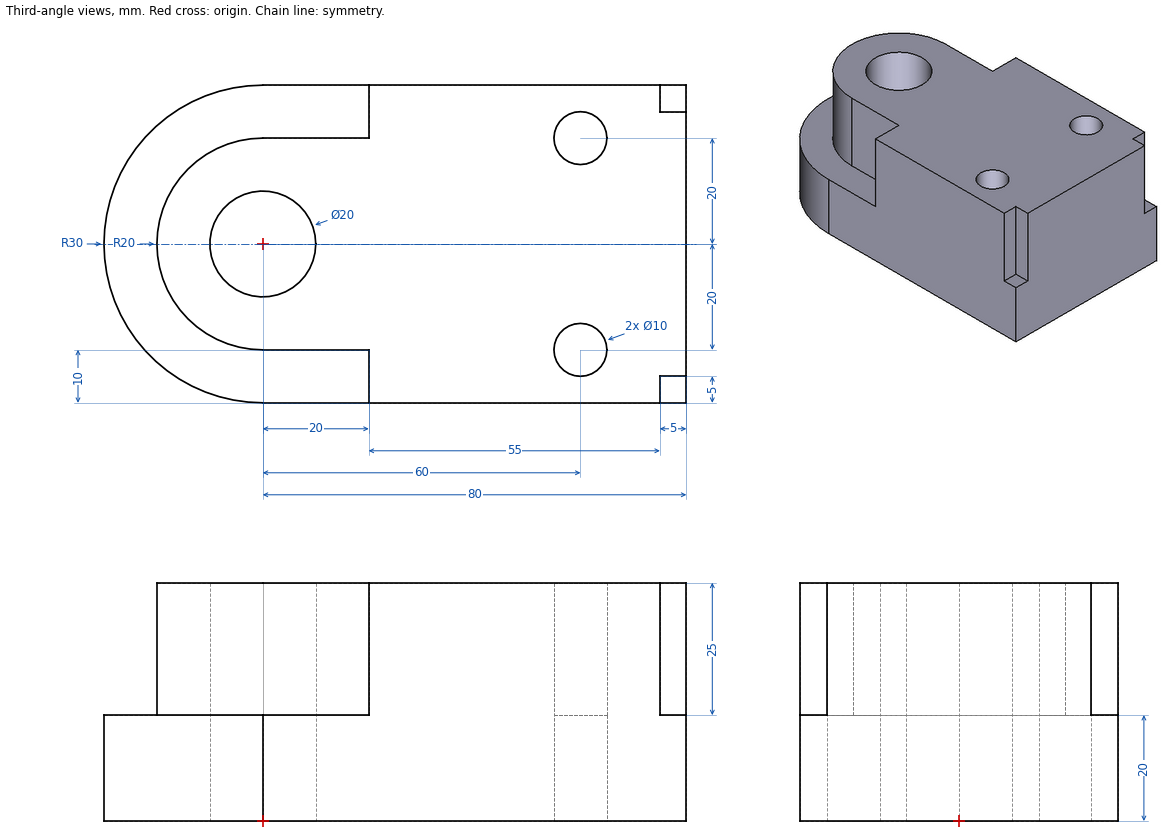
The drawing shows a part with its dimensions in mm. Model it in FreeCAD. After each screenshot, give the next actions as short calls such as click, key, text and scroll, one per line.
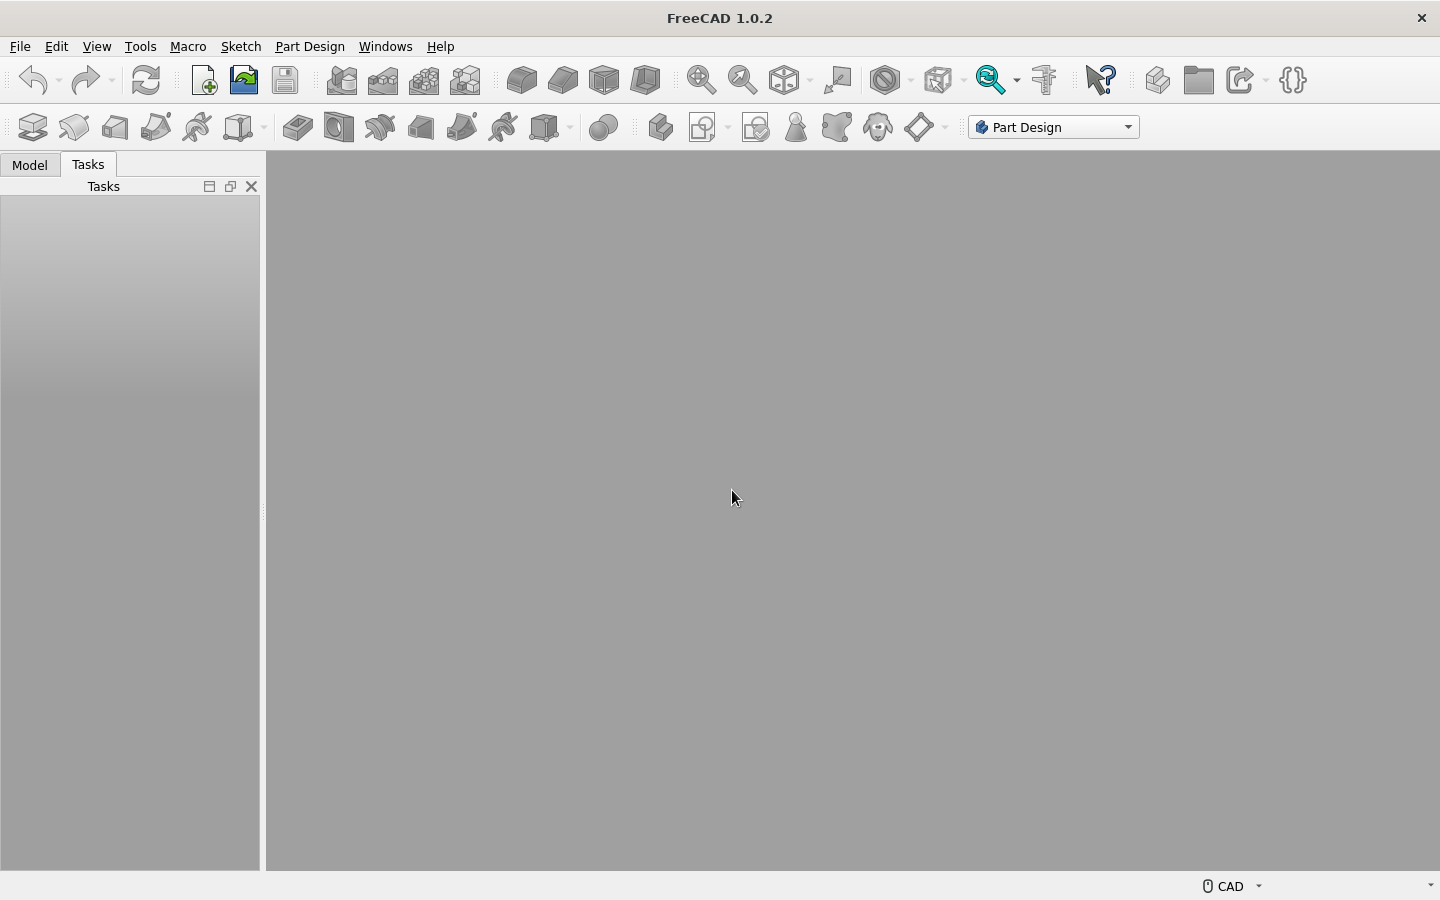
key(ctrl+n)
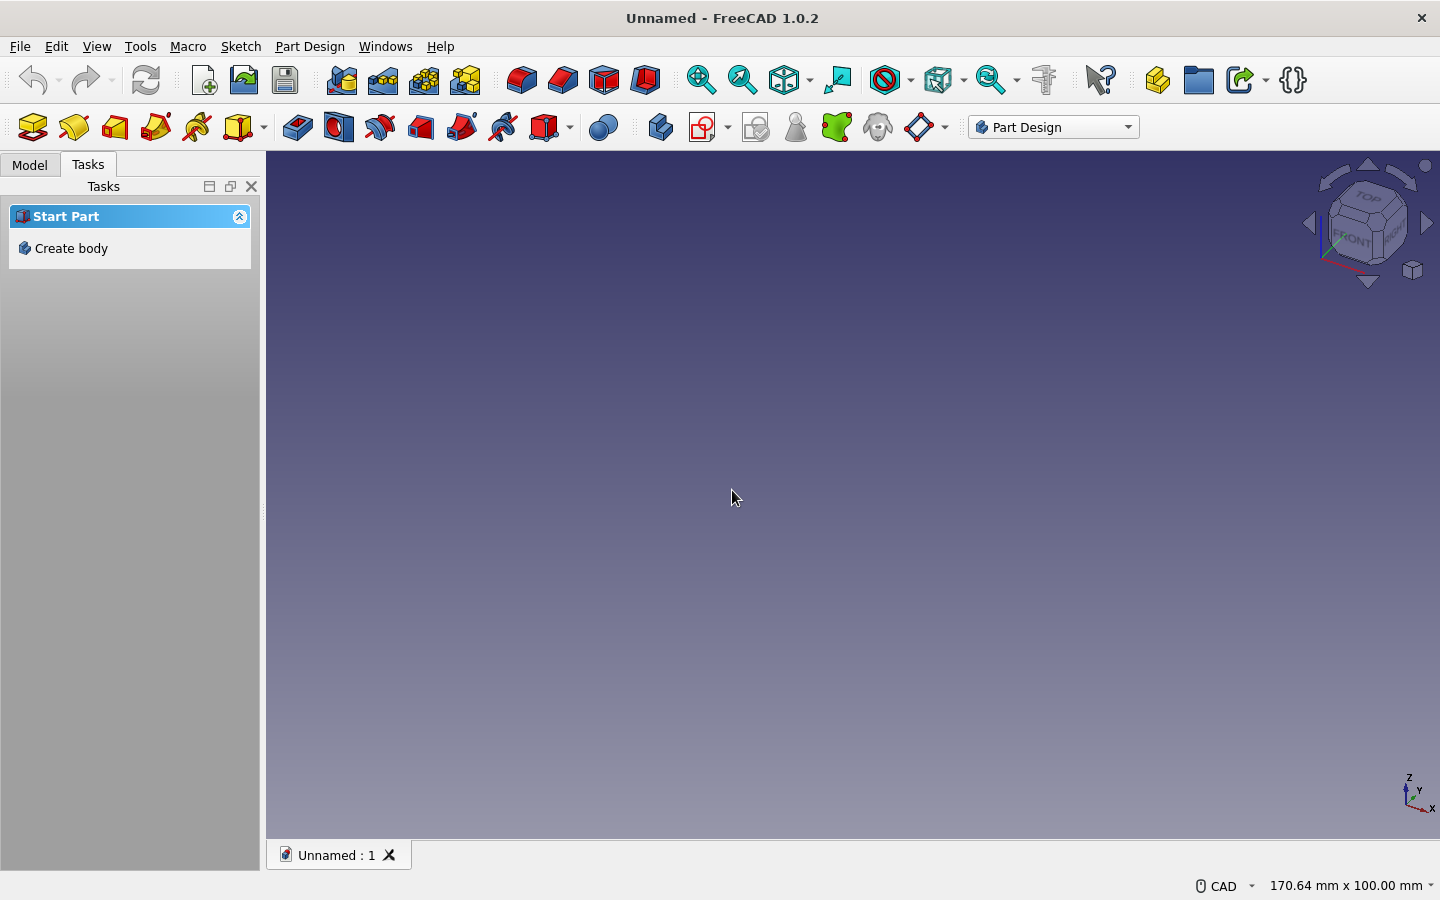
click(702, 128)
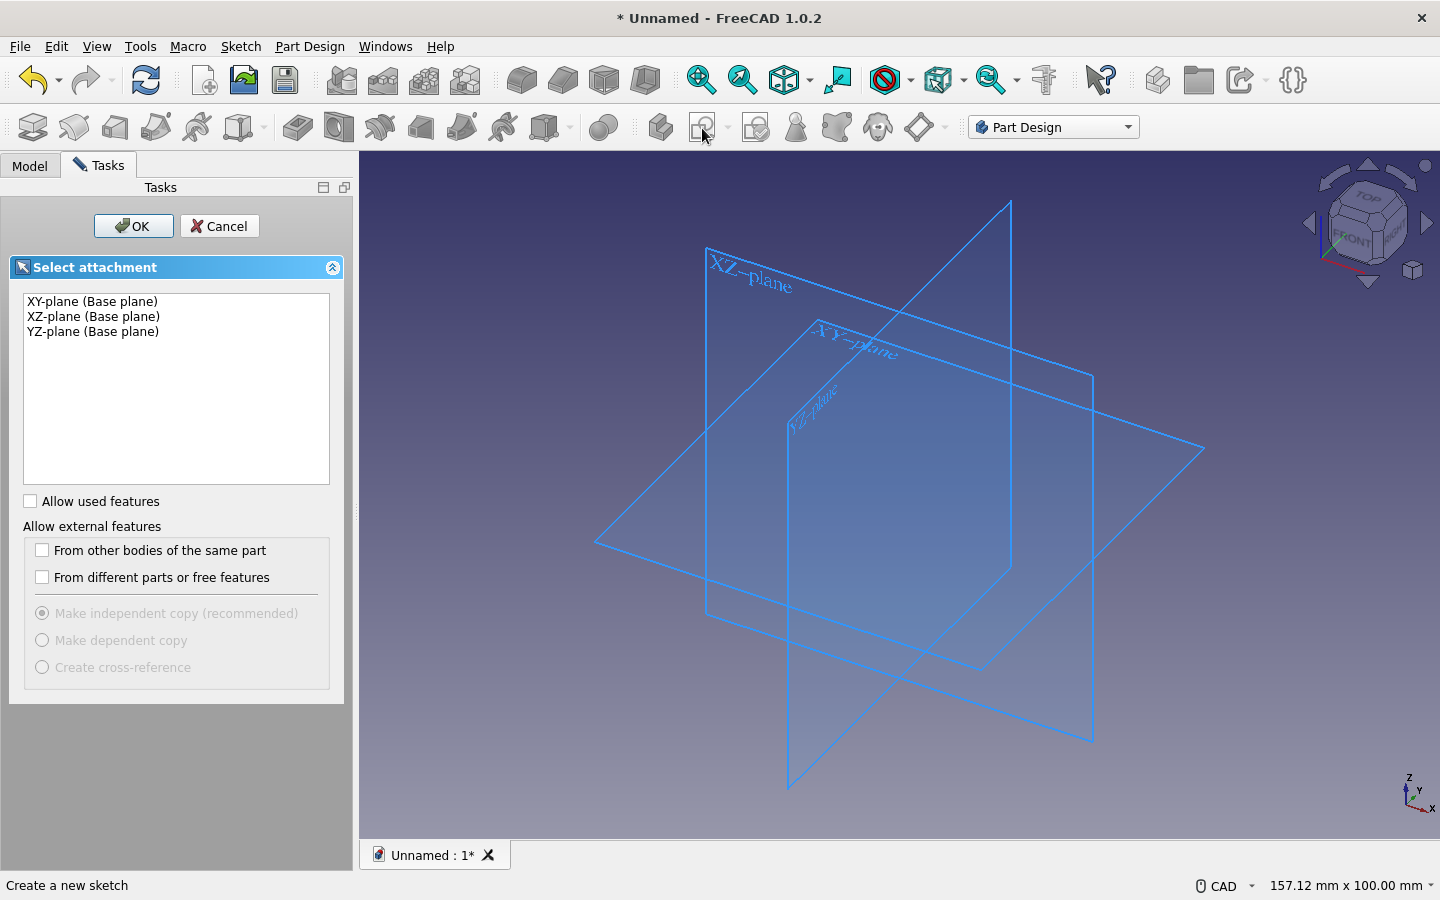
click(84, 302)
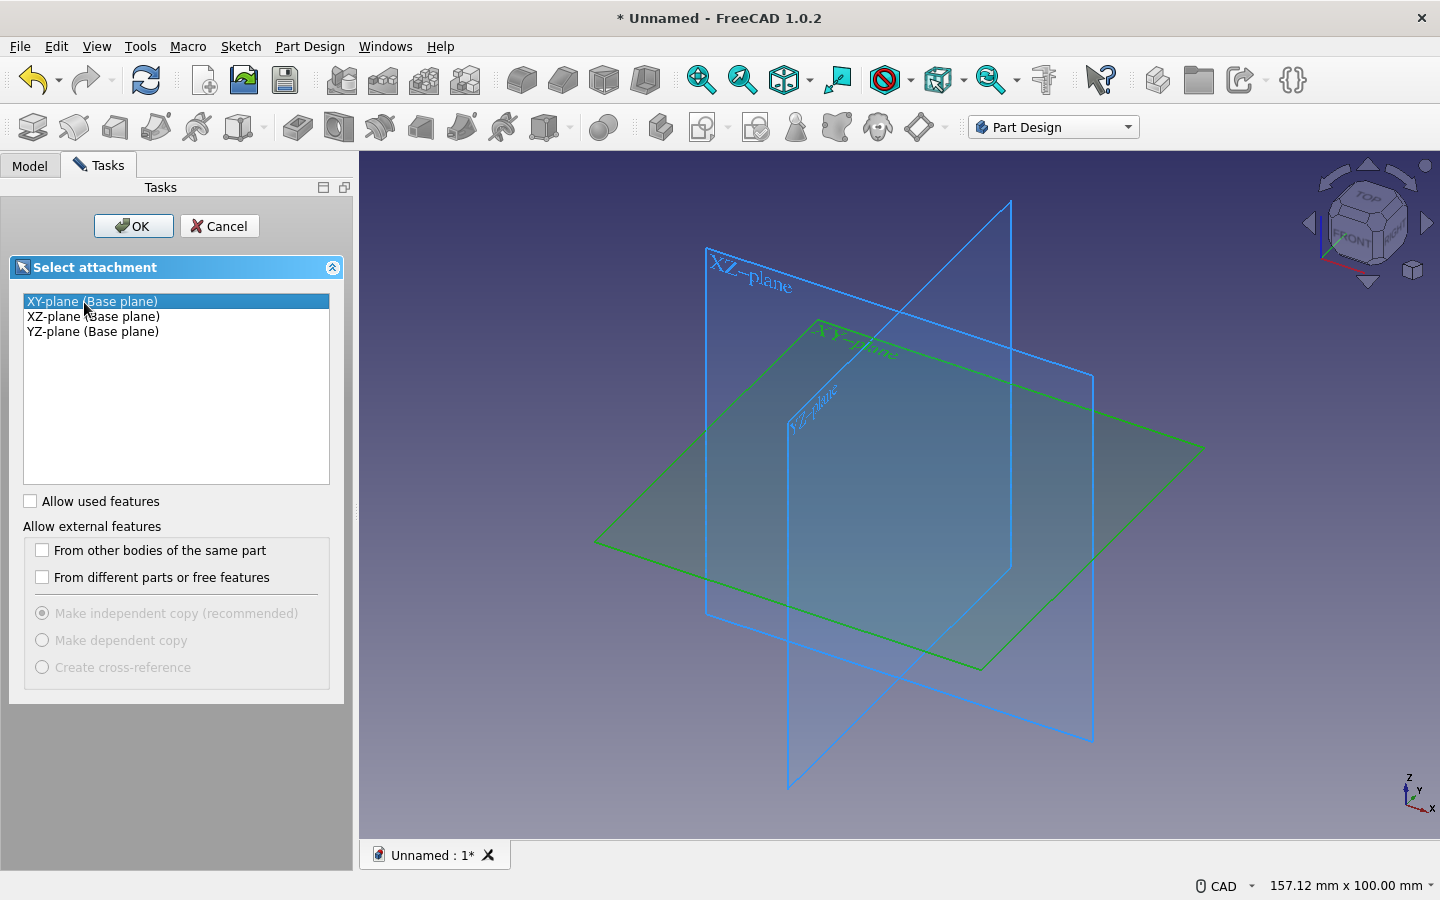
click(134, 226)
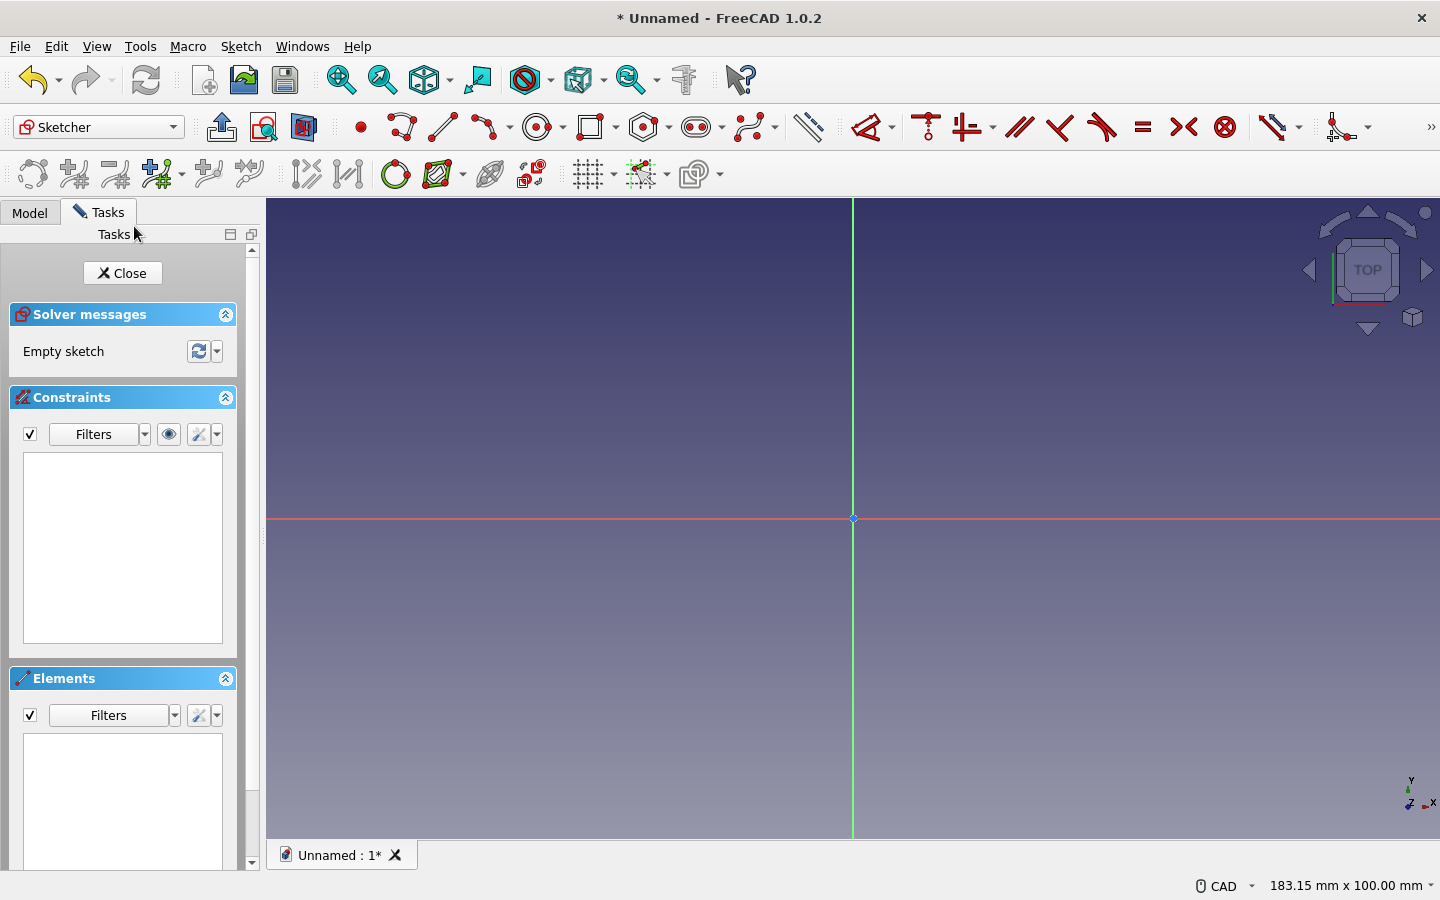
scroll(294, 519, down, 1)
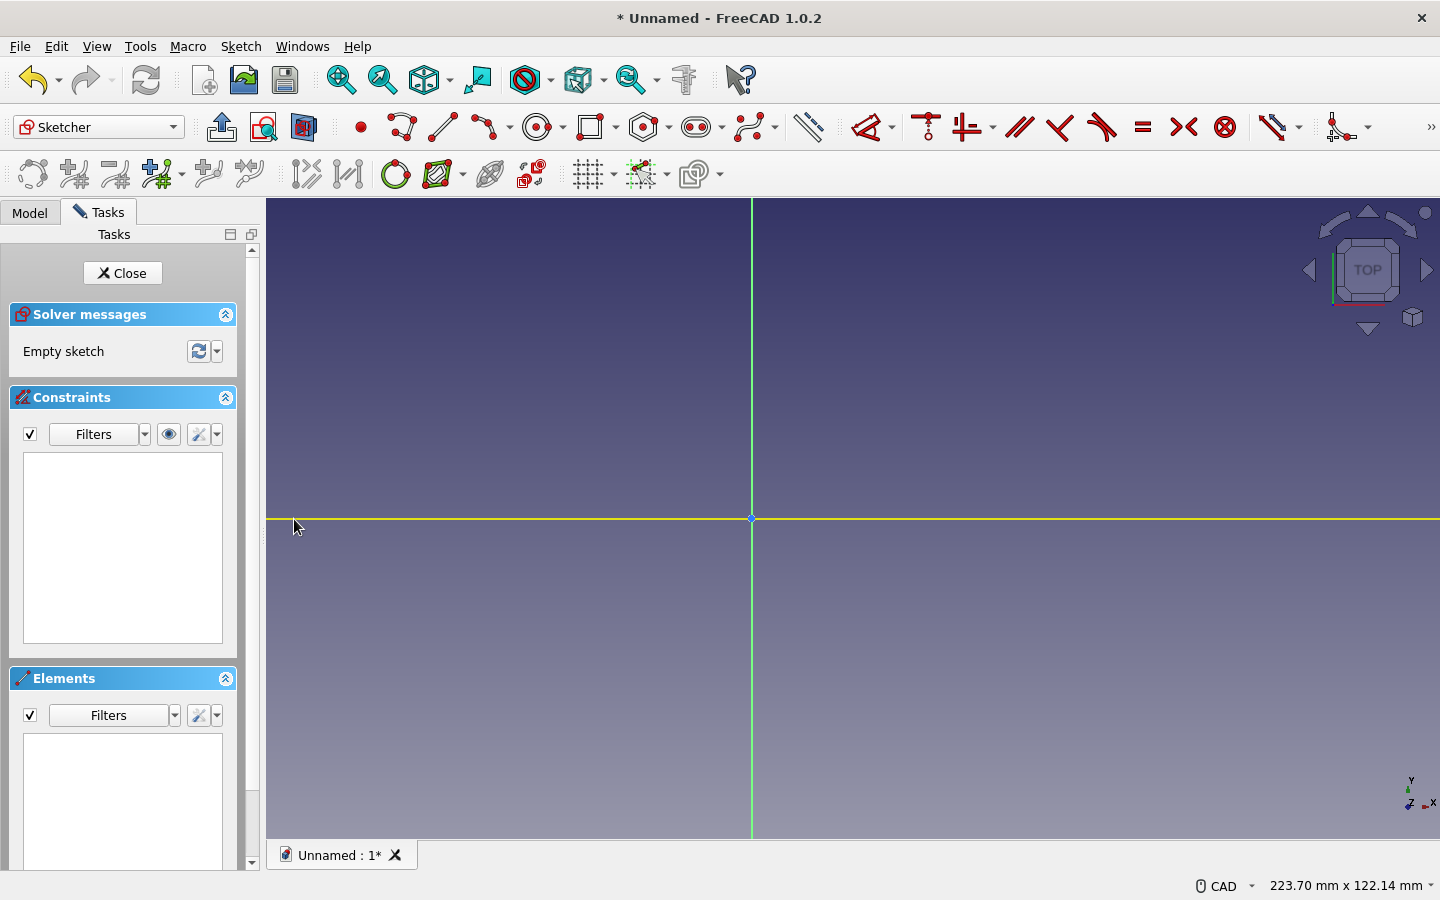
click(402, 128)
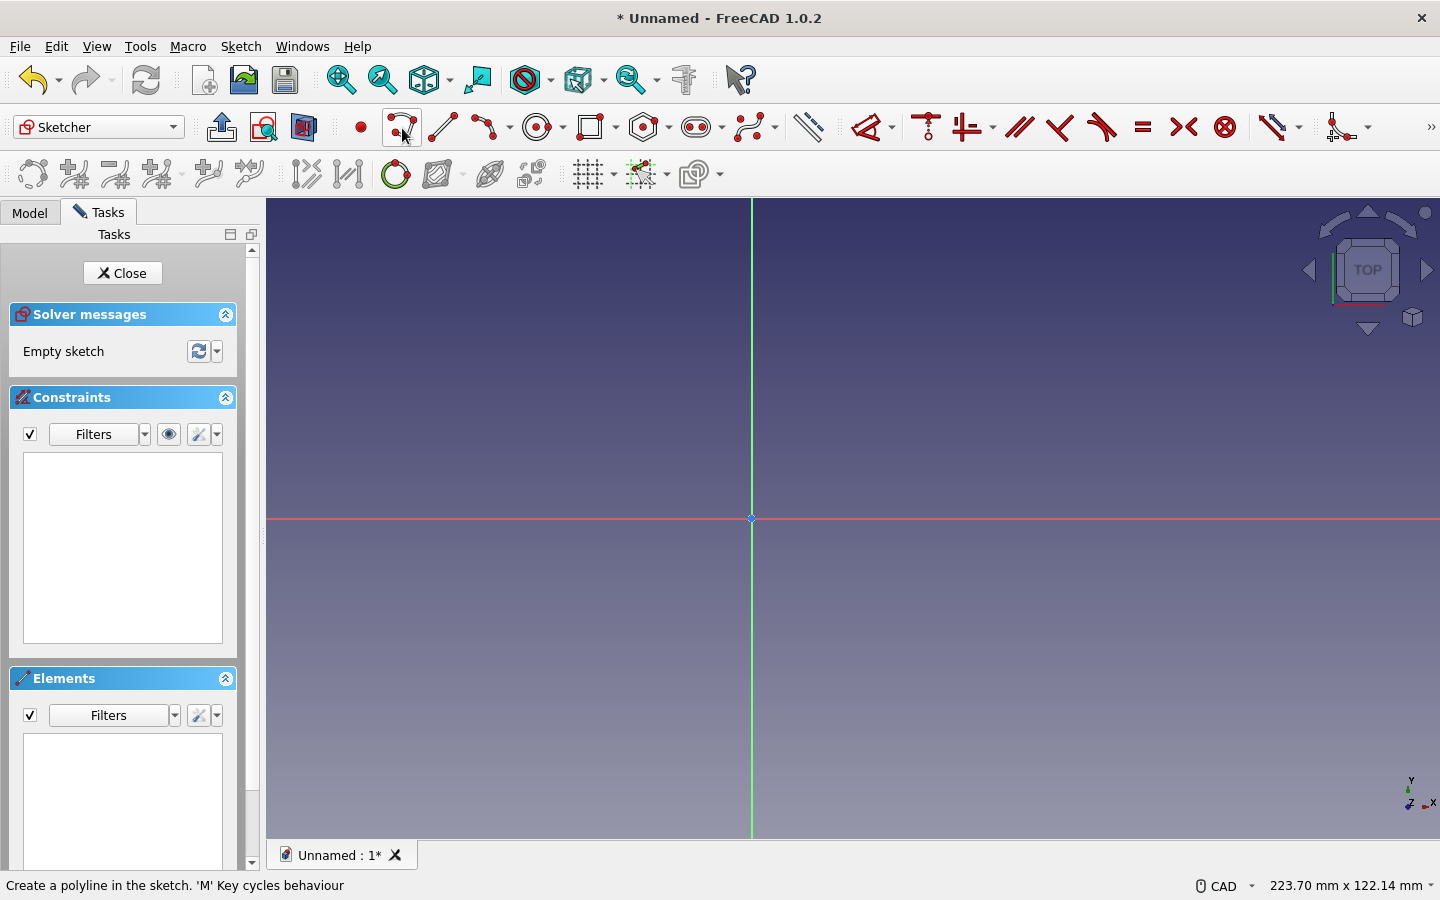
click(752, 676)
click(1172, 676)
click(1172, 361)
click(752, 361)
right_click(752, 361)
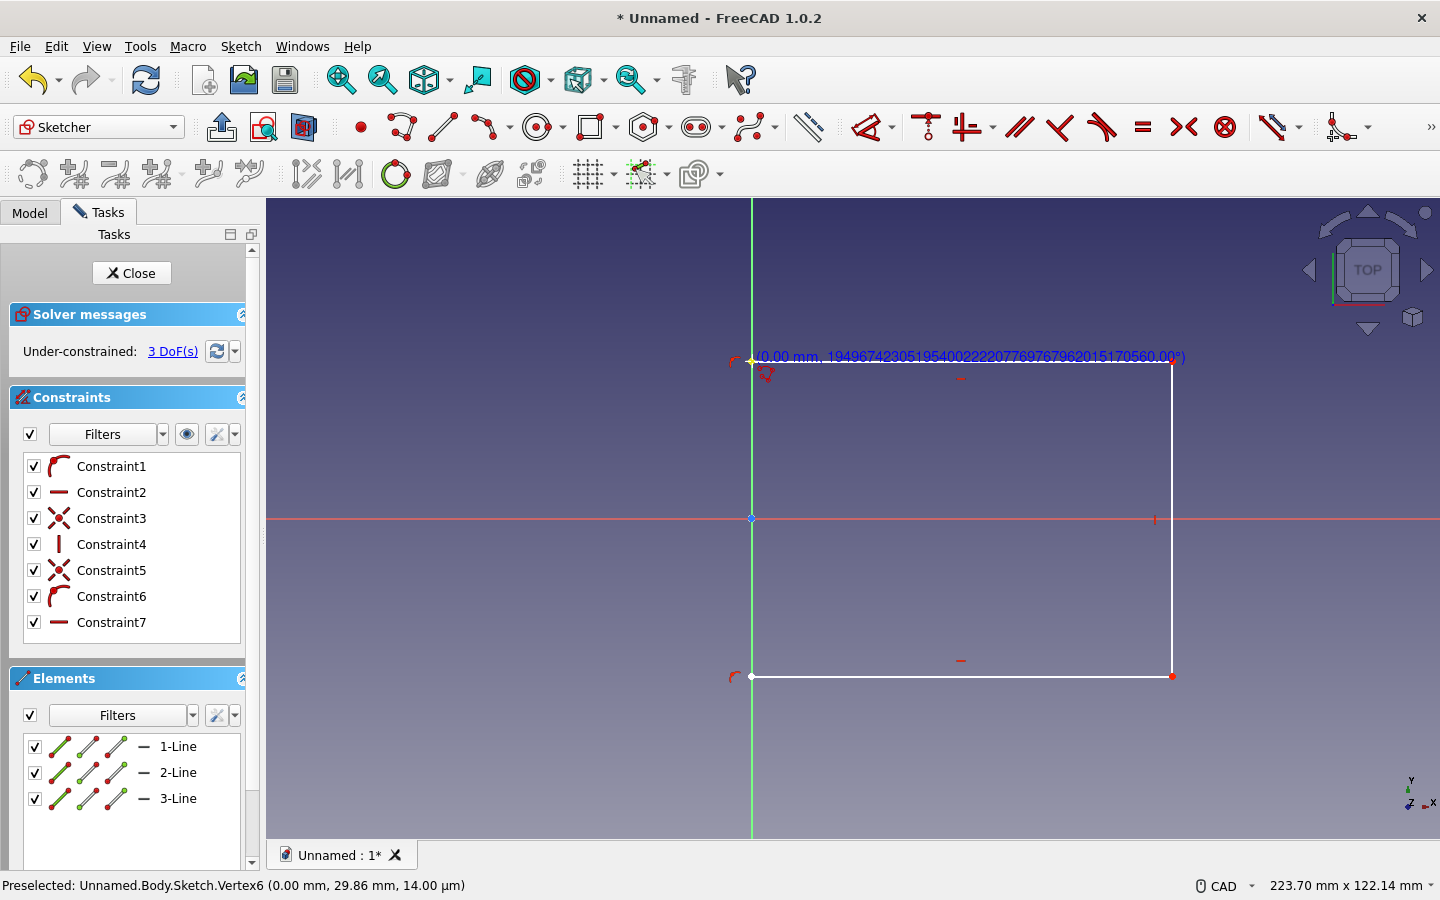
click(484, 128)